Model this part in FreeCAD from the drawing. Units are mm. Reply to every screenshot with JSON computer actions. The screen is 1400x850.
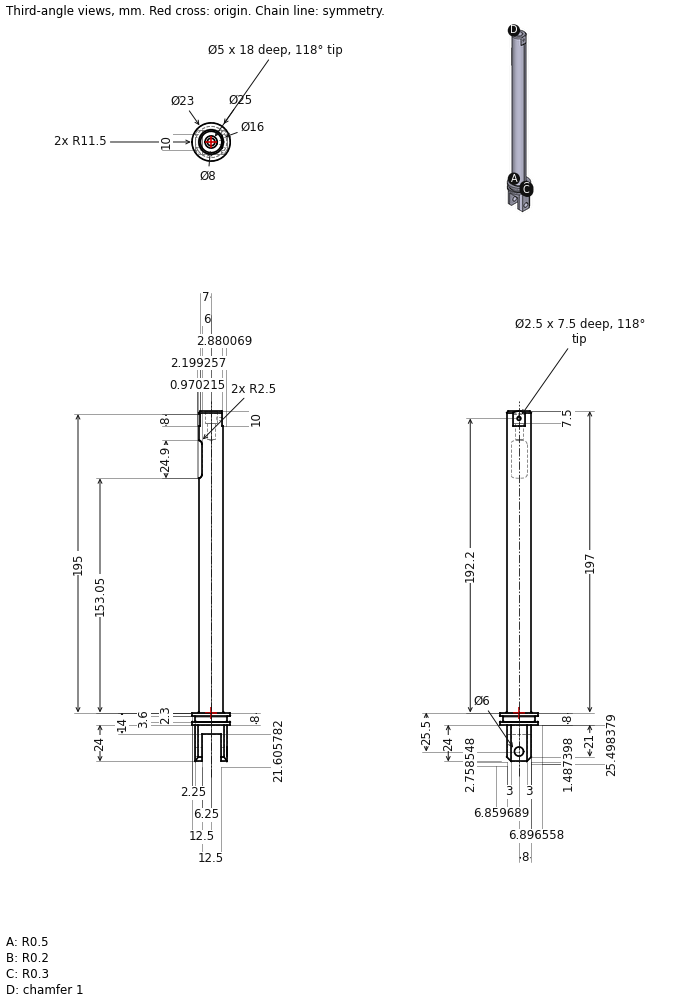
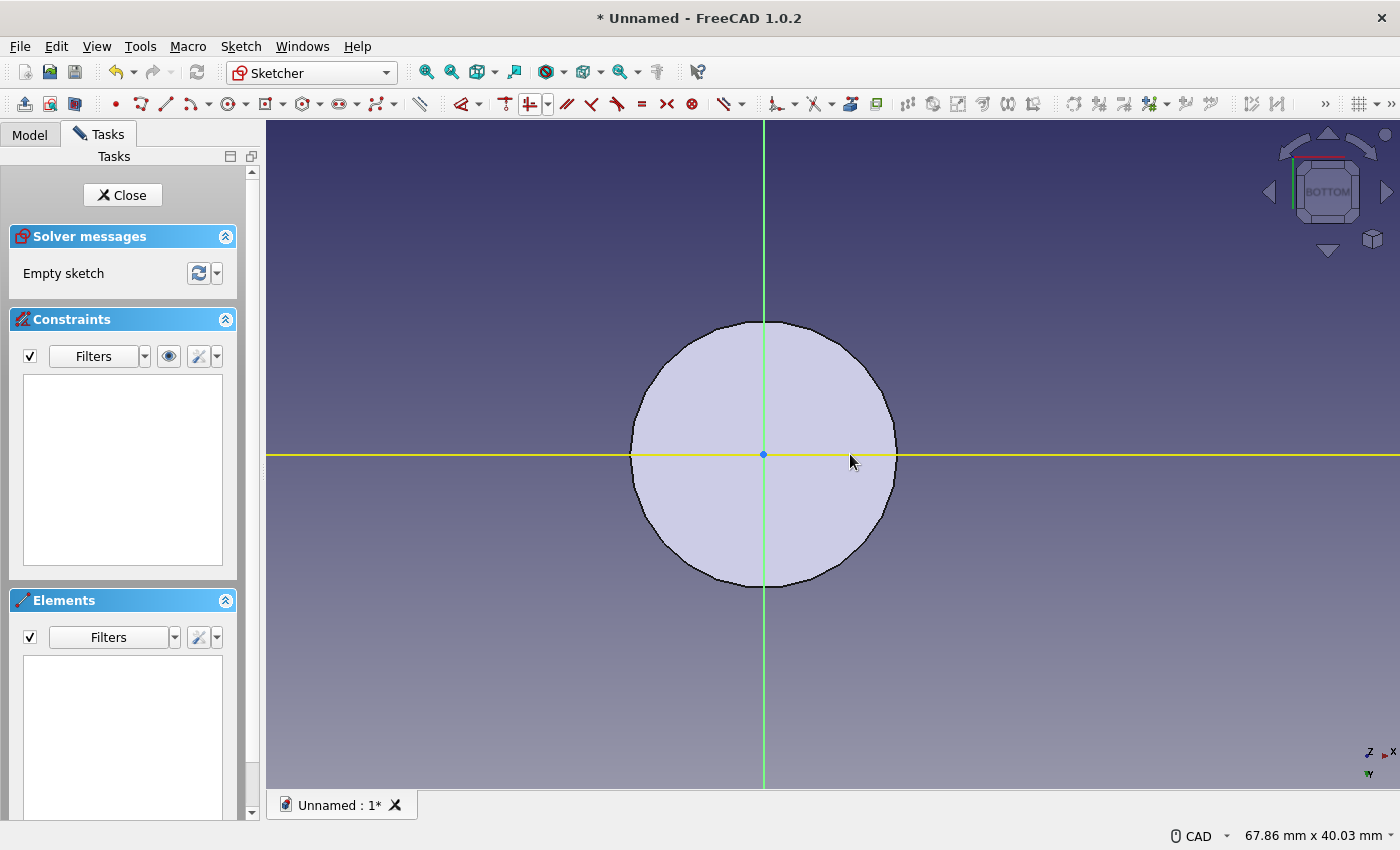
{"action": "left_click", "coordinate": [228, 104]}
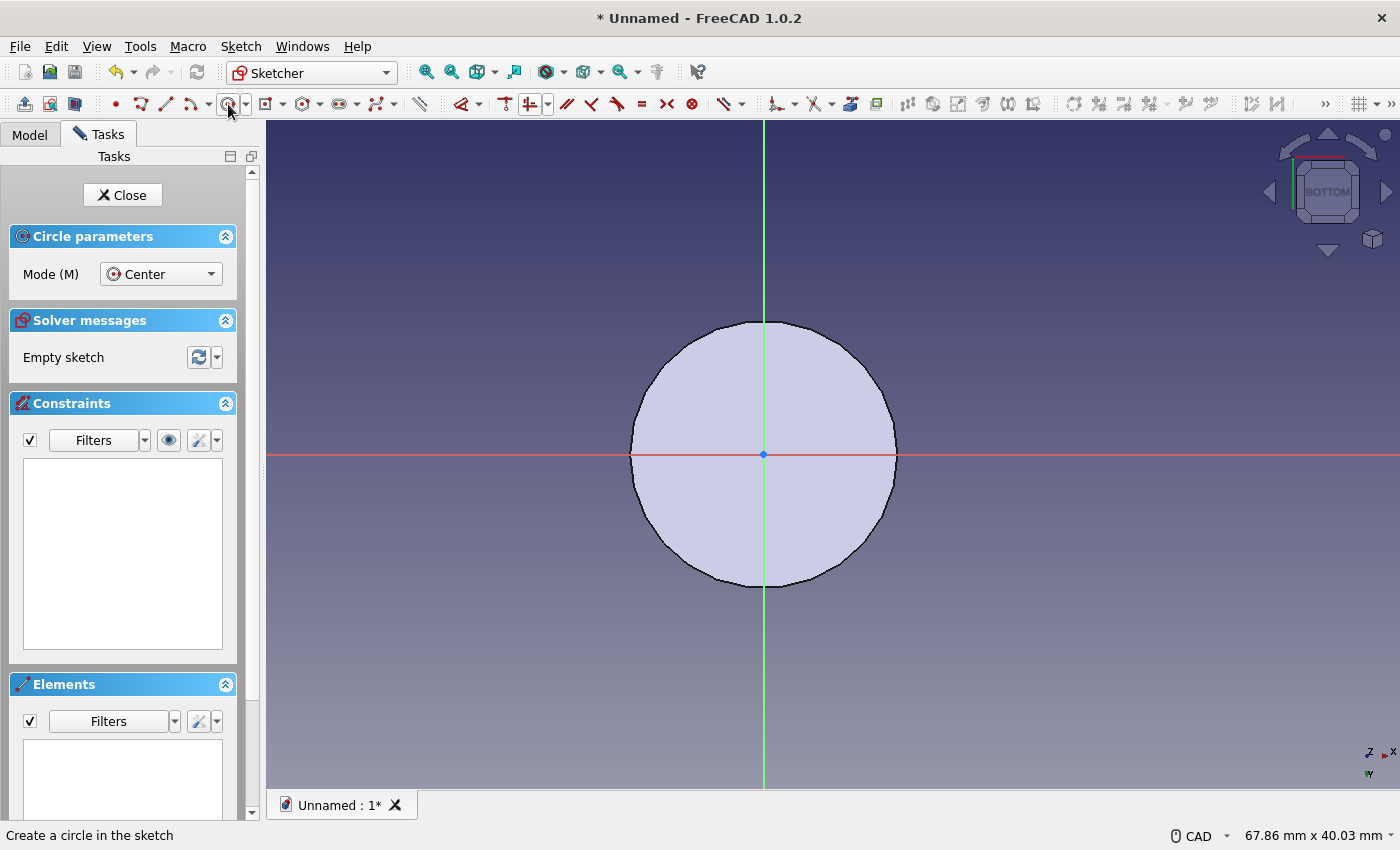
{"action": "left_click", "coordinate": [764, 454]}
{"action": "mouse_move", "coordinate": [911, 307]}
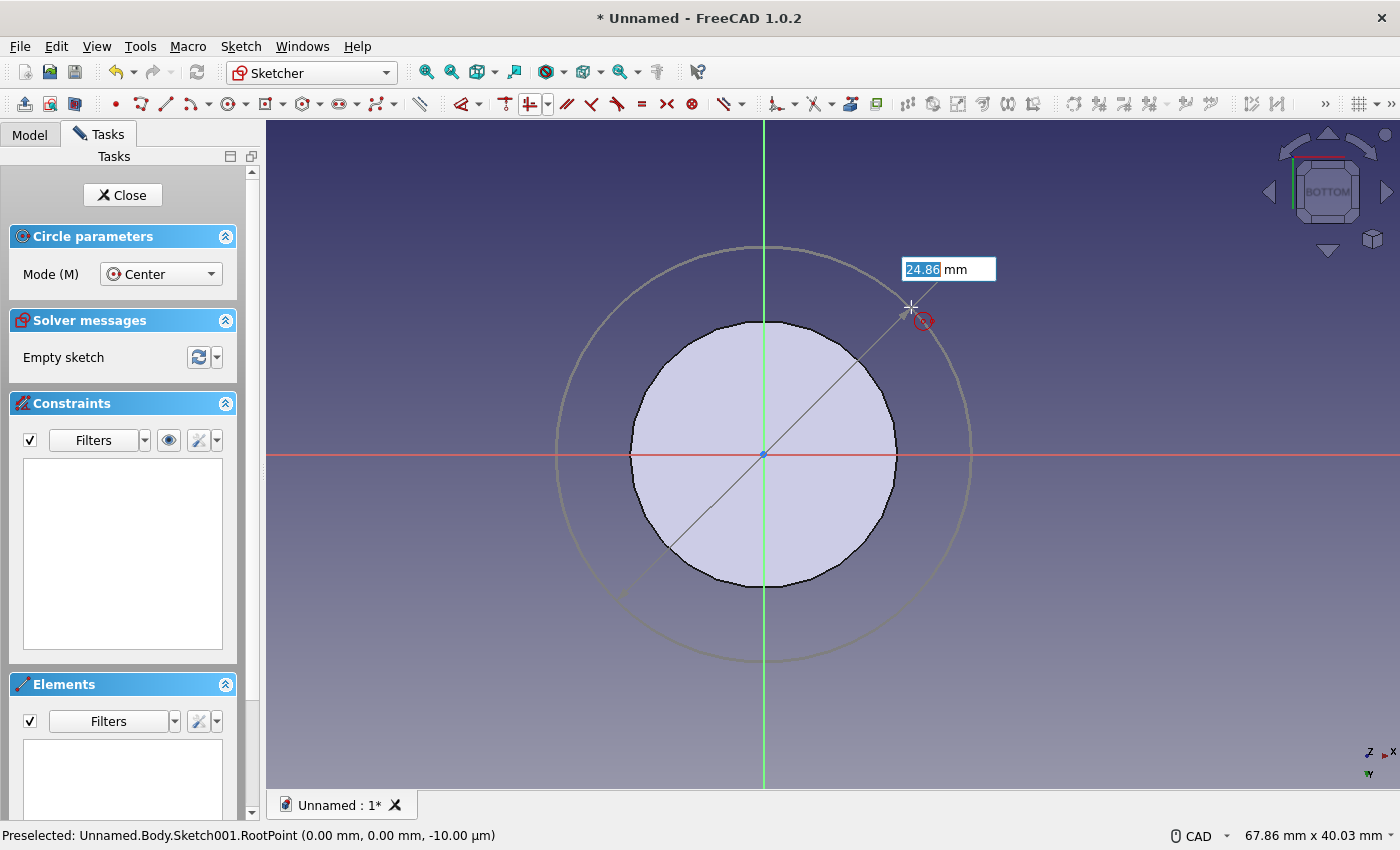
{"action": "type", "text": "25"}
{"action": "key", "text": "Return"}
{"action": "key", "text": "Escape"}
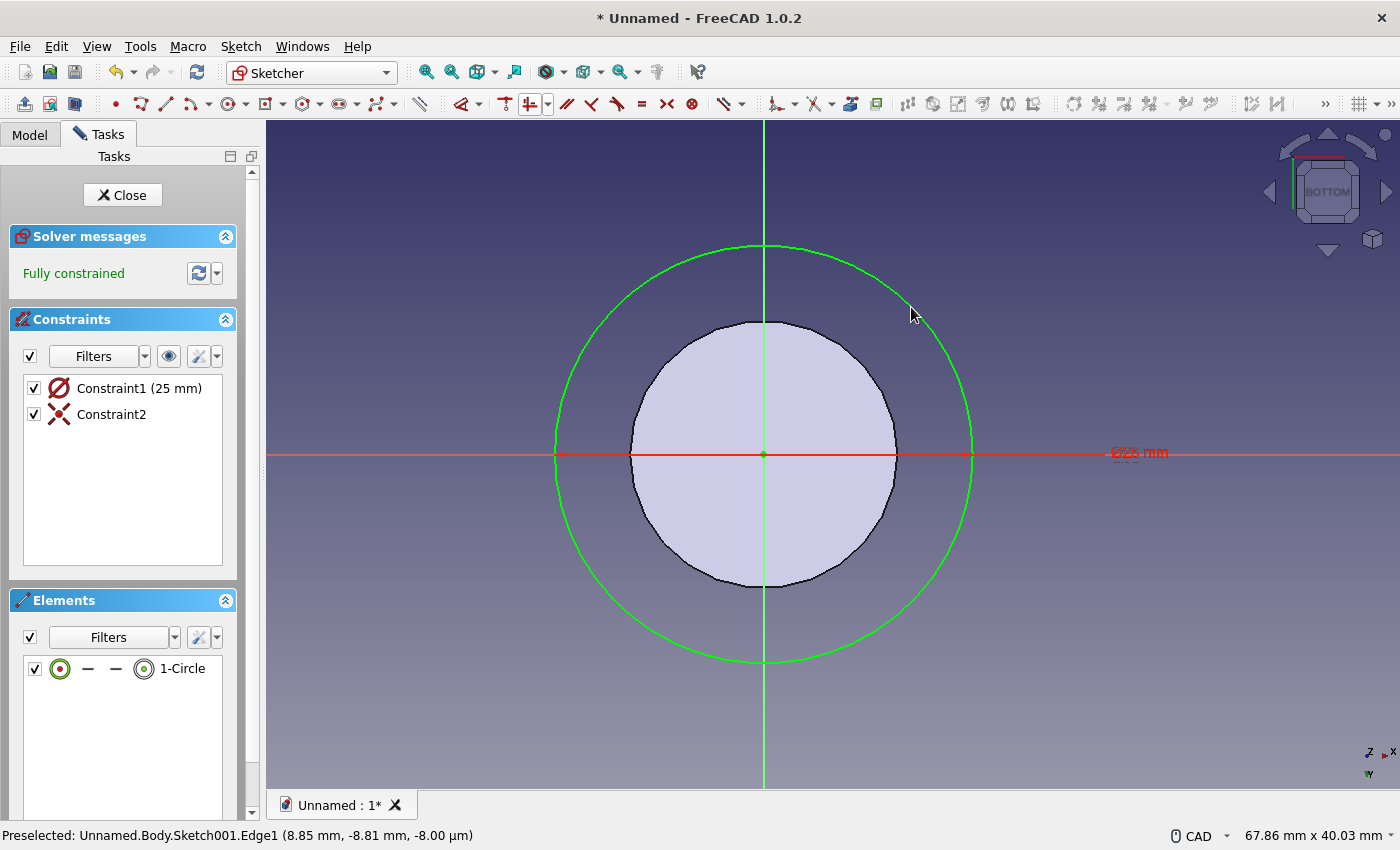
{"action": "left_click", "coordinate": [123, 195]}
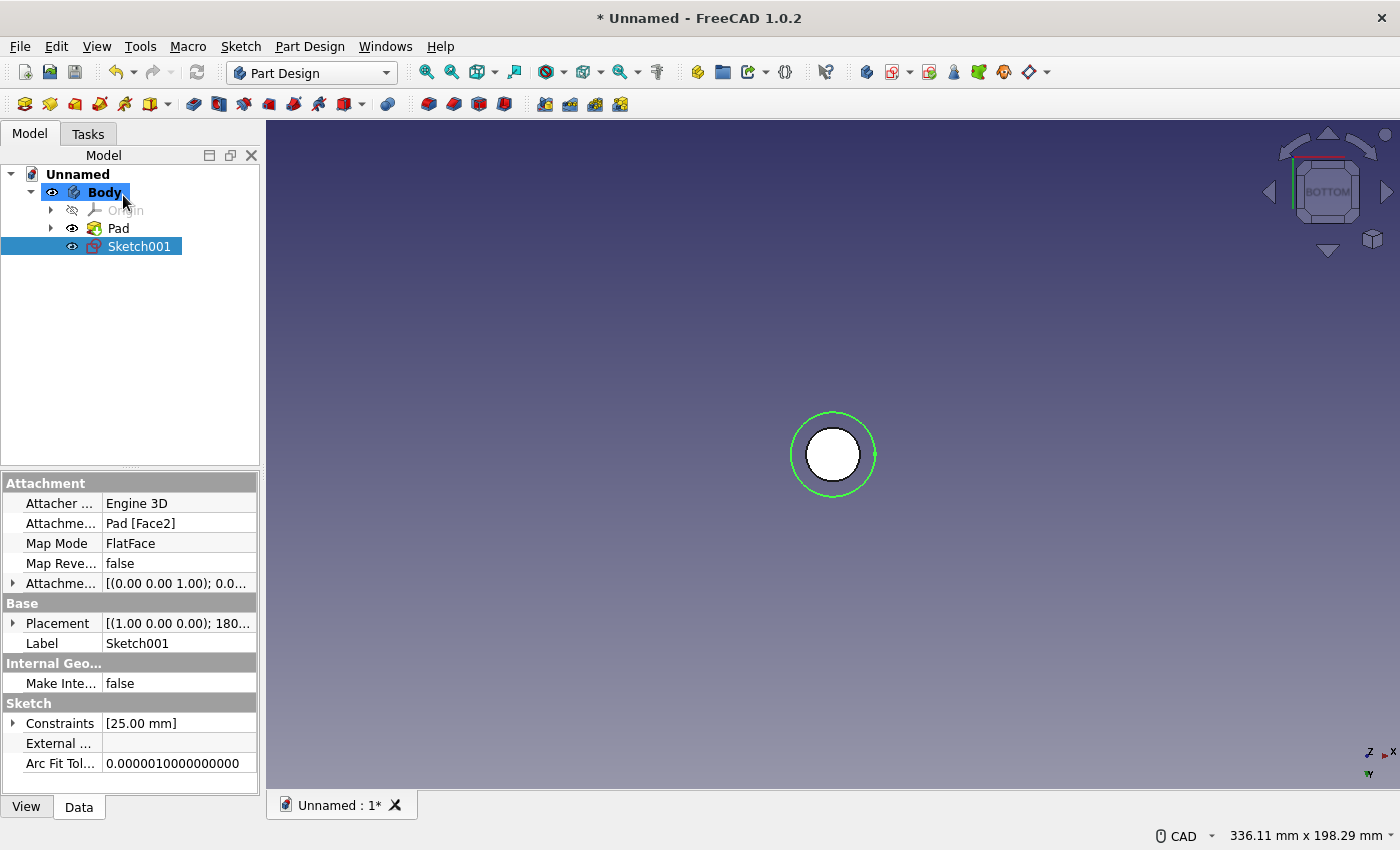
{"action": "left_click", "coordinate": [25, 104]}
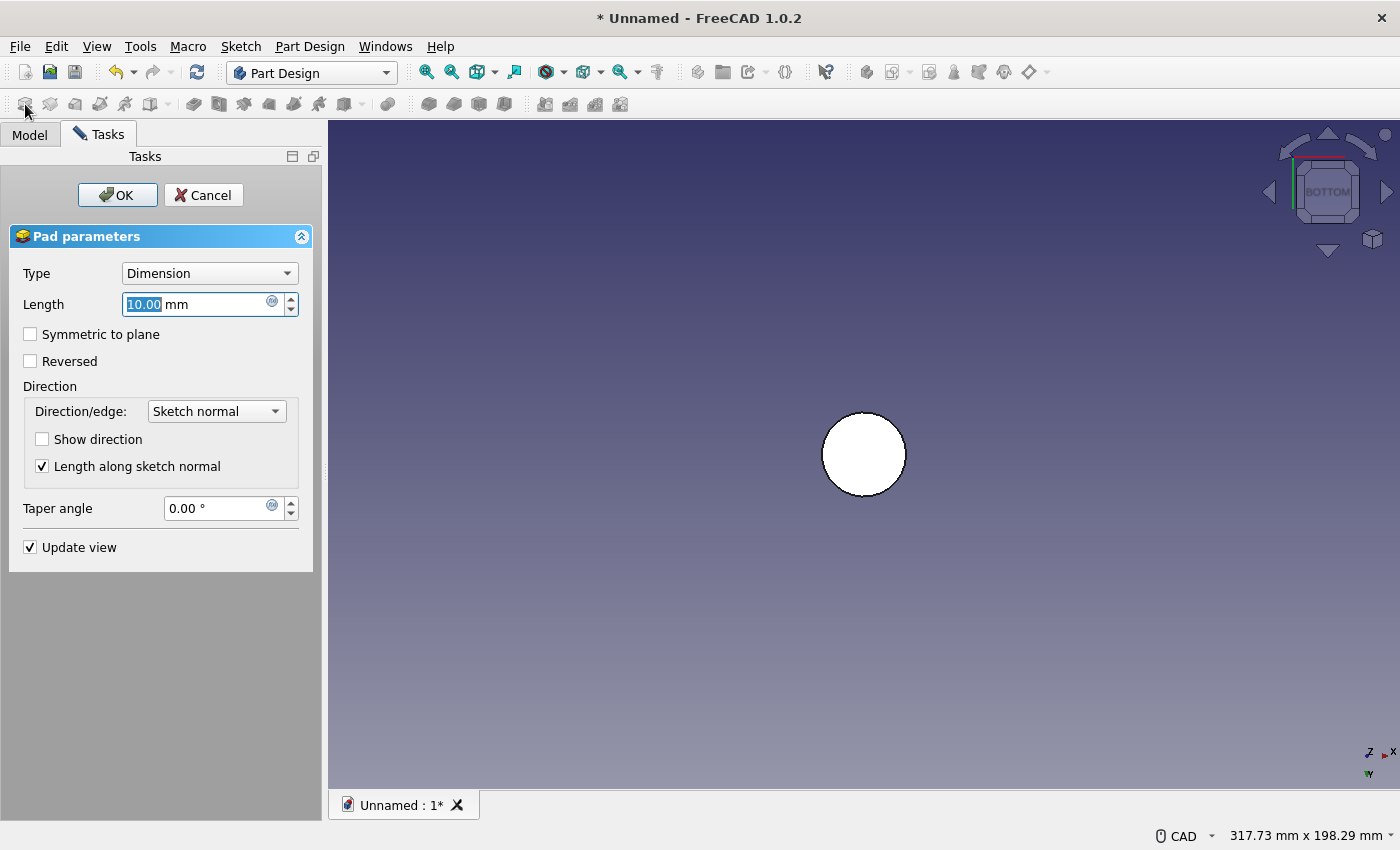
{"action": "type", "text": "8"}
{"action": "key", "text": "Tab"}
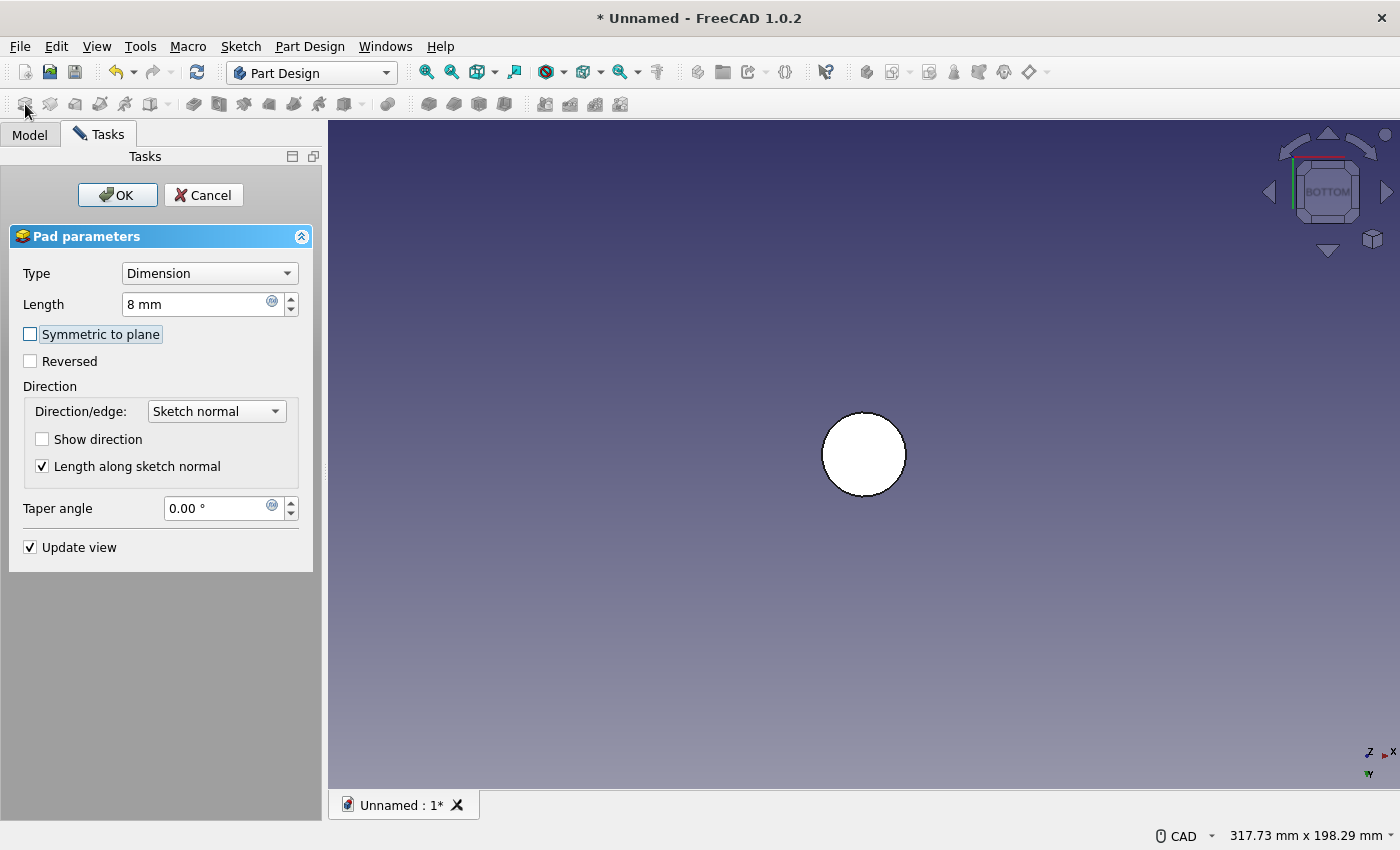
{"action": "left_click", "coordinate": [118, 195]}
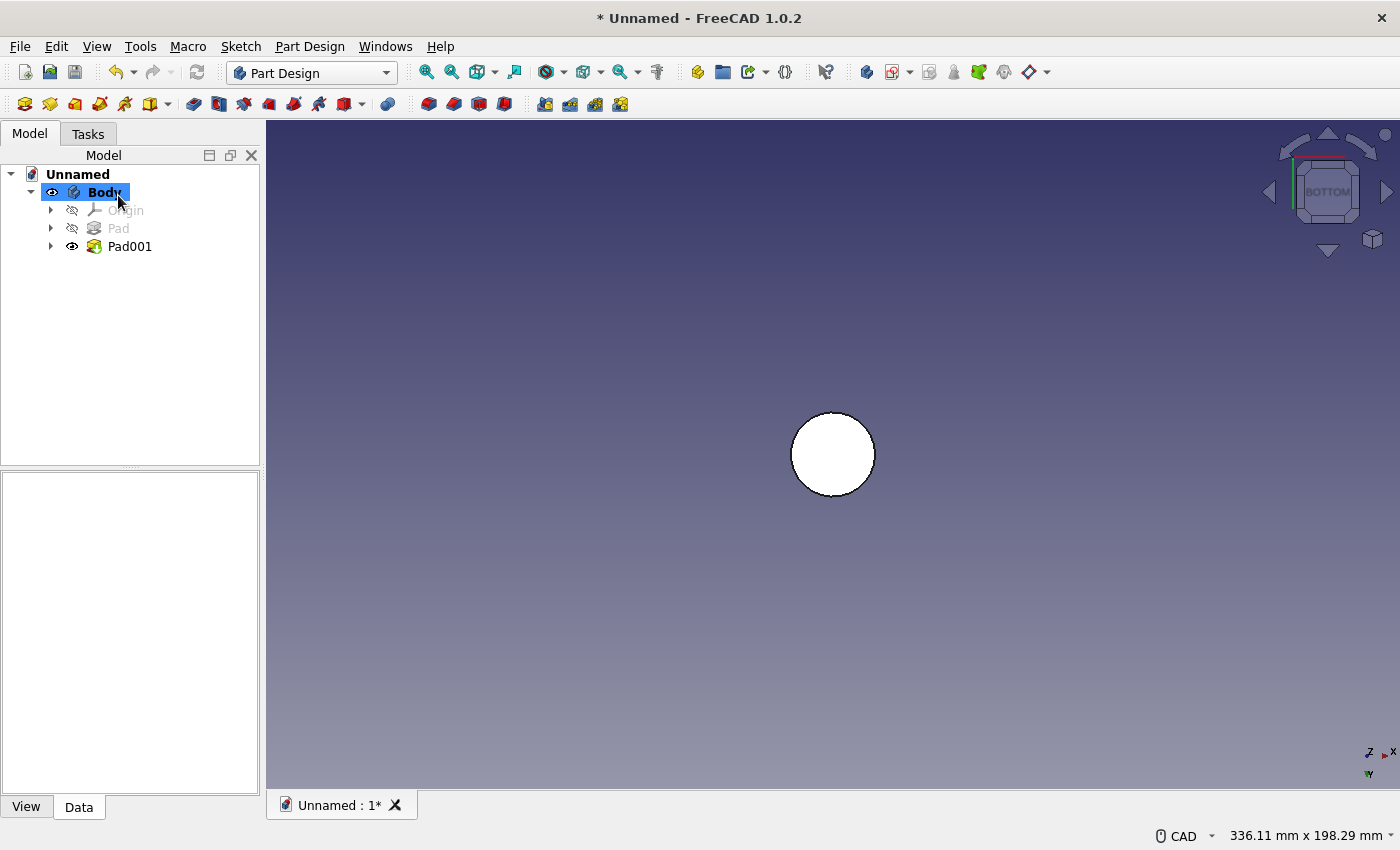
{"action": "left_click", "coordinate": [427, 72]}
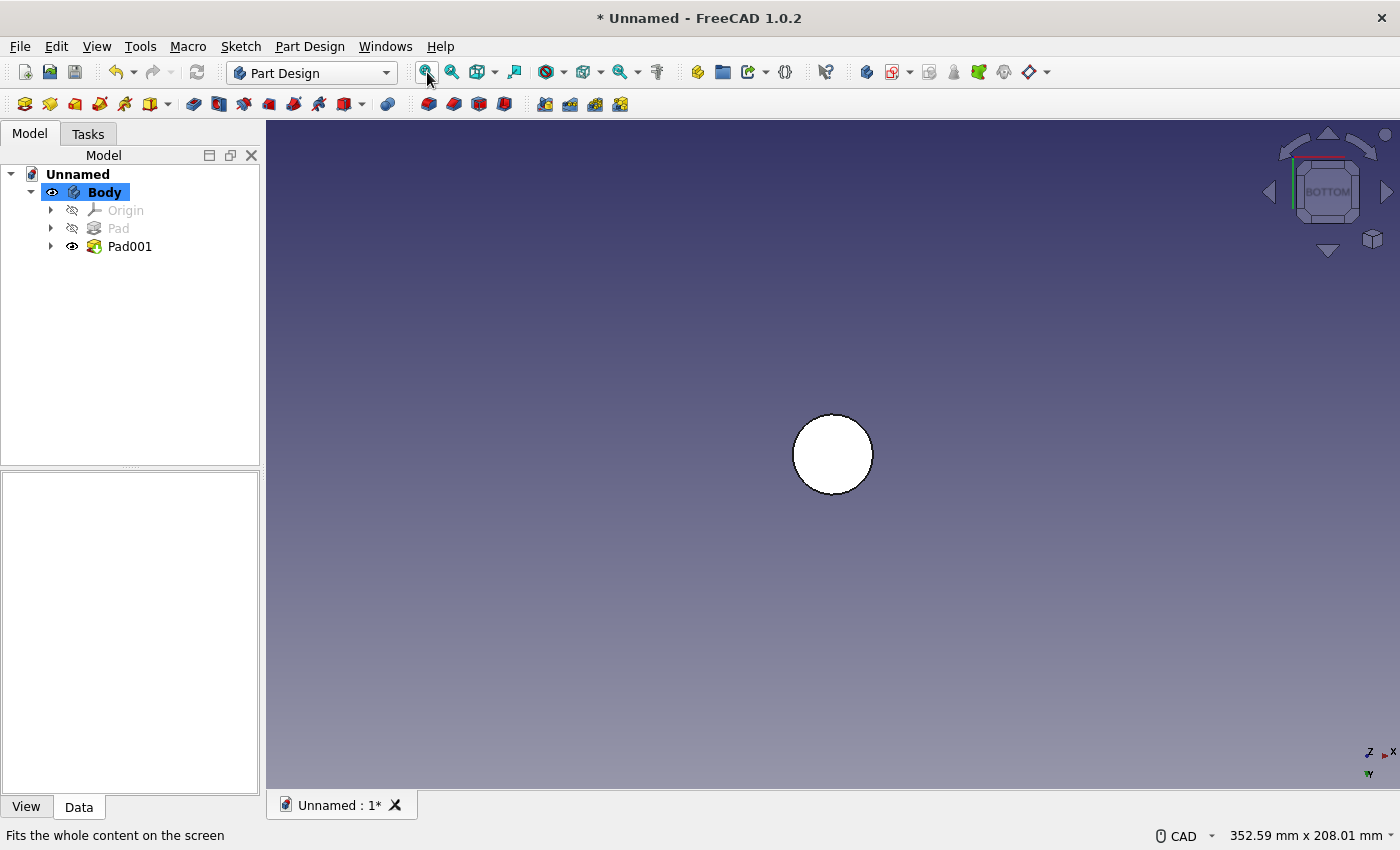
{"action": "left_click", "coordinate": [892, 72]}